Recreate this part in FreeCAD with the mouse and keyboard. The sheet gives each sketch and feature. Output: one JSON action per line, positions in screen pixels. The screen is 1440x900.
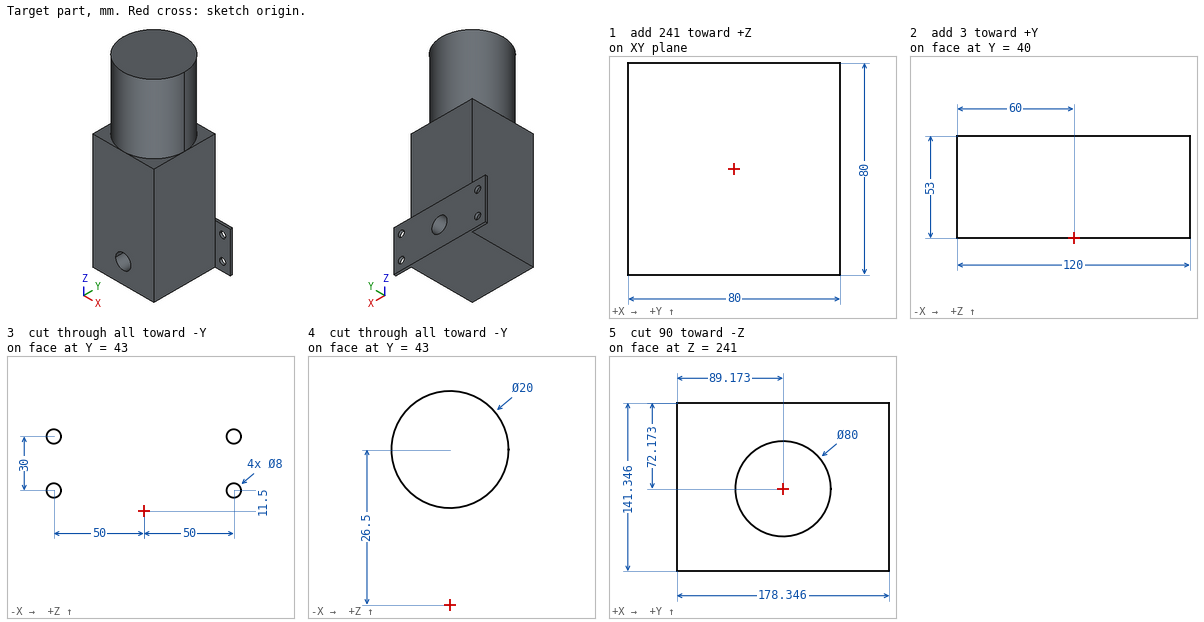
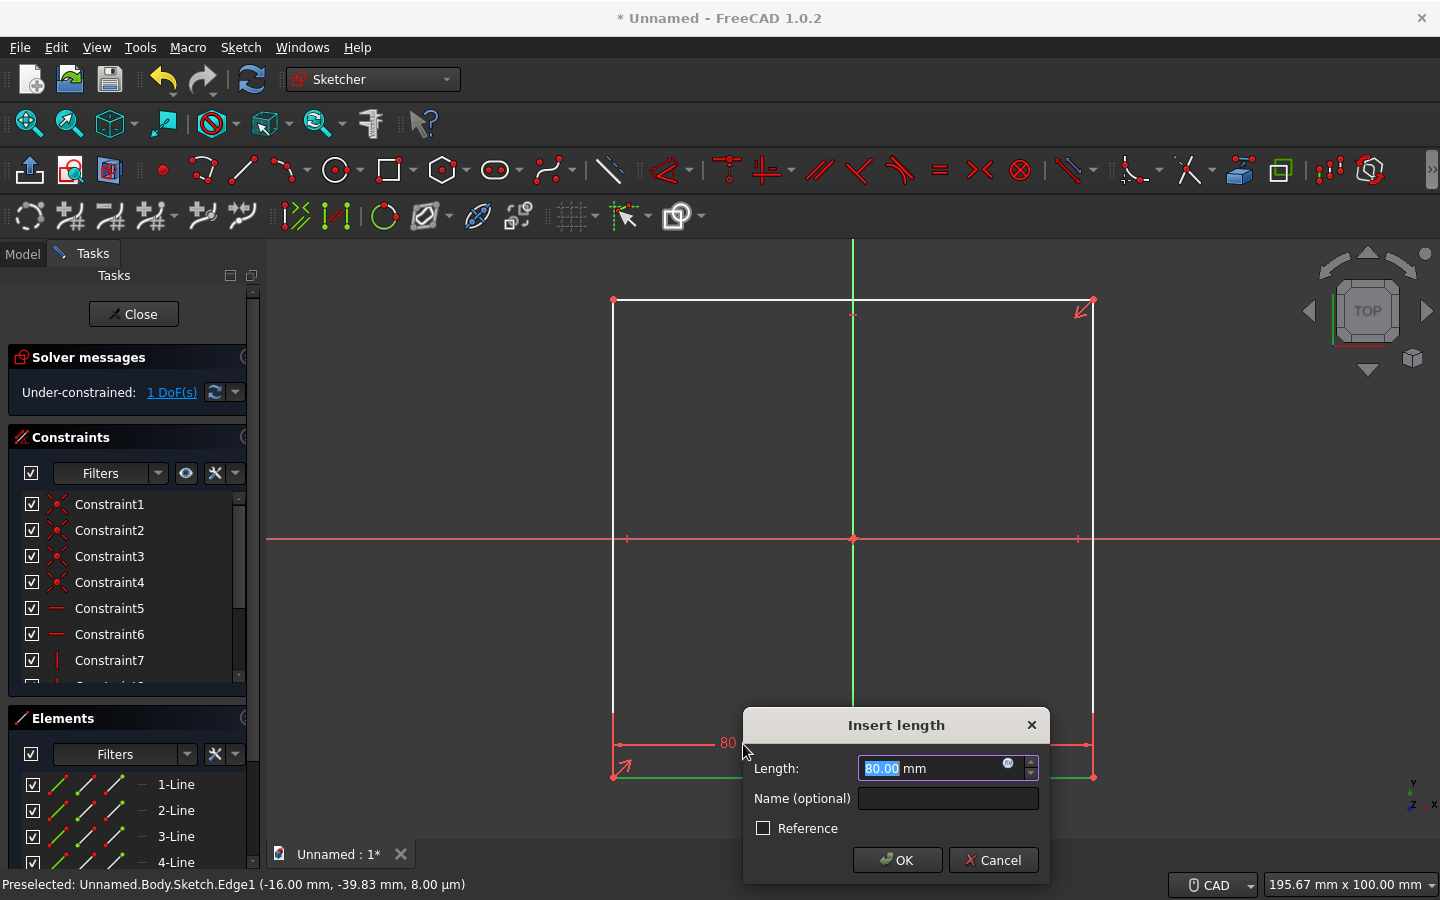
{"action": "type", "text": "80"}
{"action": "key", "text": "Return"}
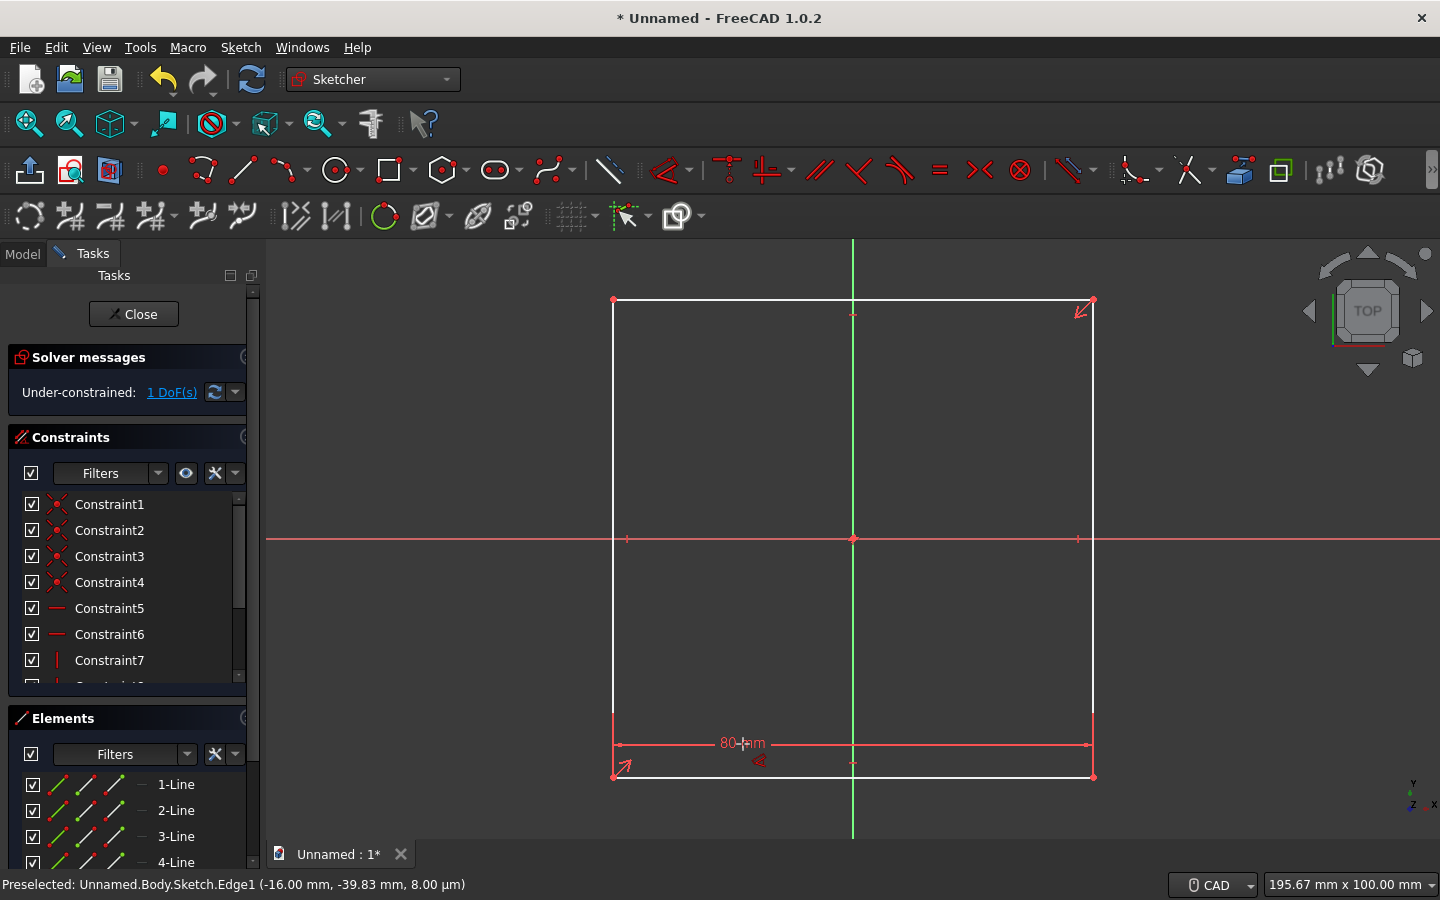
{"action": "left_click", "coordinate": [1093, 635]}
{"action": "left_click", "coordinate": [1127, 429]}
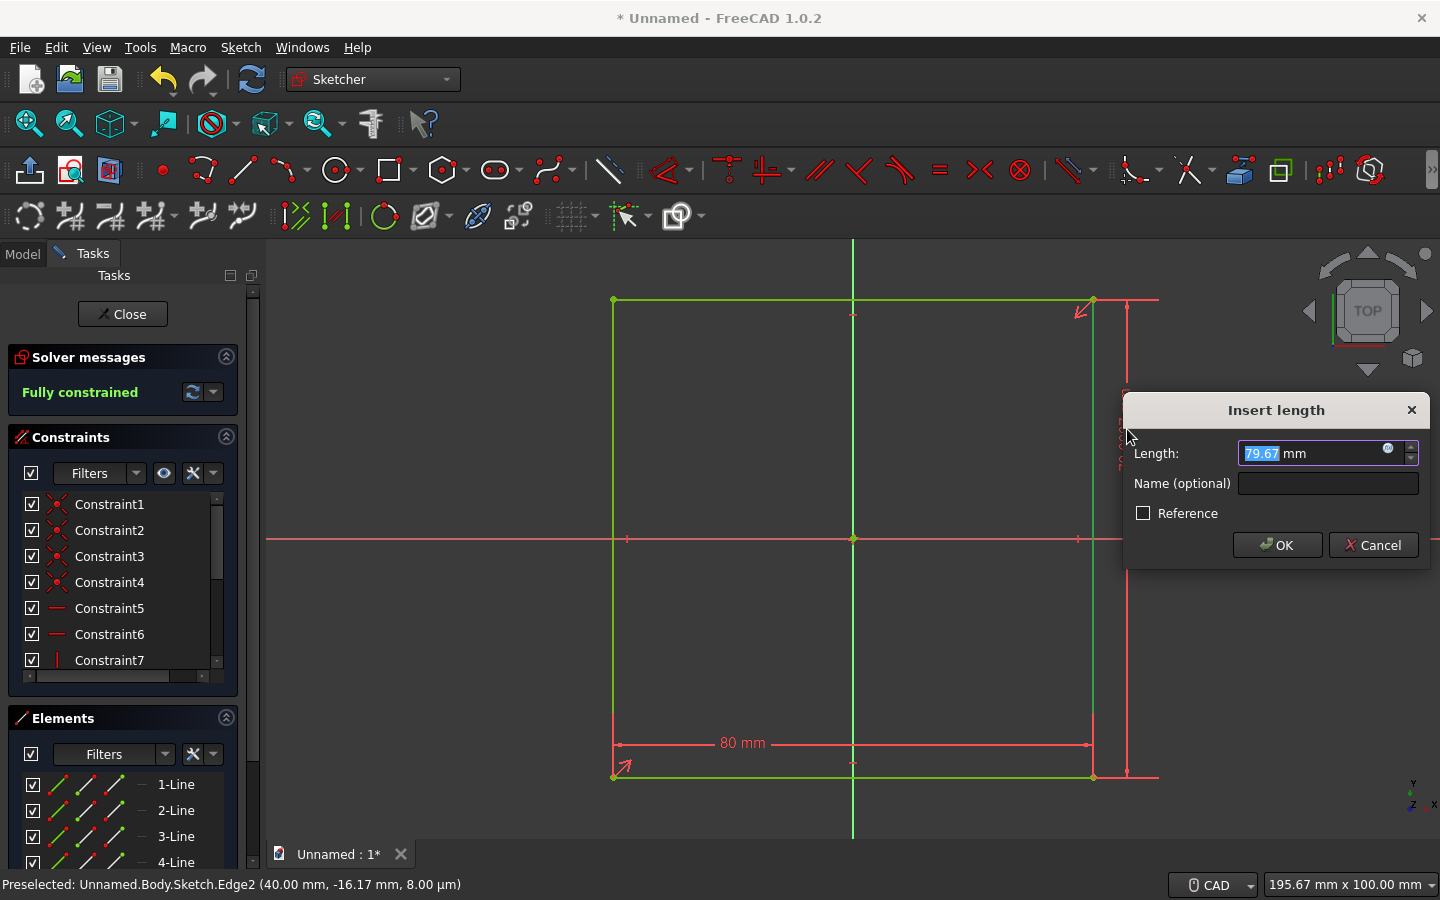
{"action": "type", "text": "80"}
{"action": "key", "text": "Return"}
{"action": "key", "text": "Escape"}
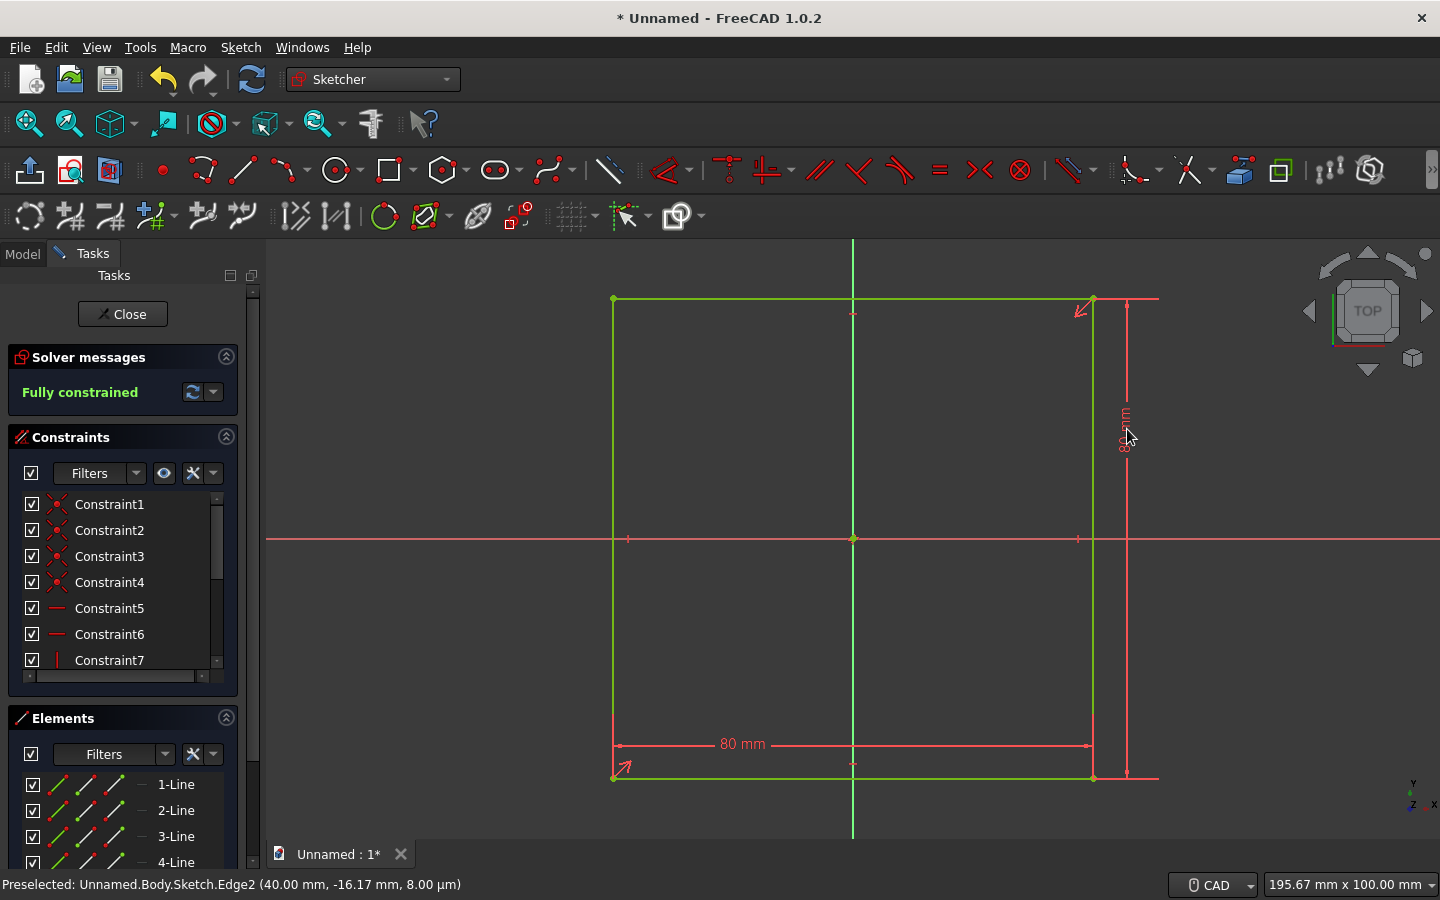
{"action": "left_click", "coordinate": [123, 314]}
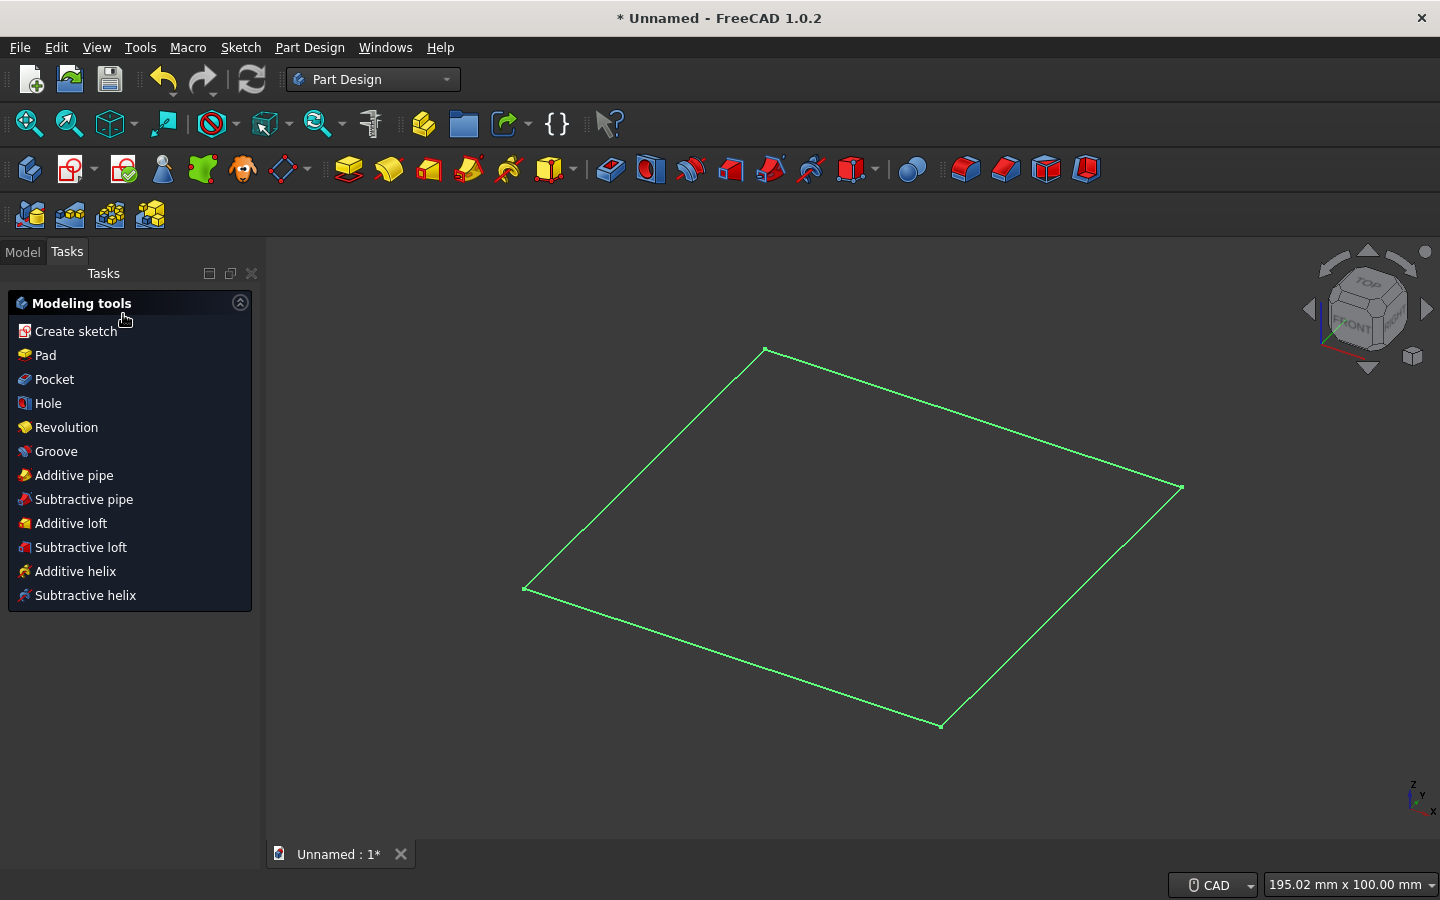
{"action": "left_click", "coordinate": [350, 170]}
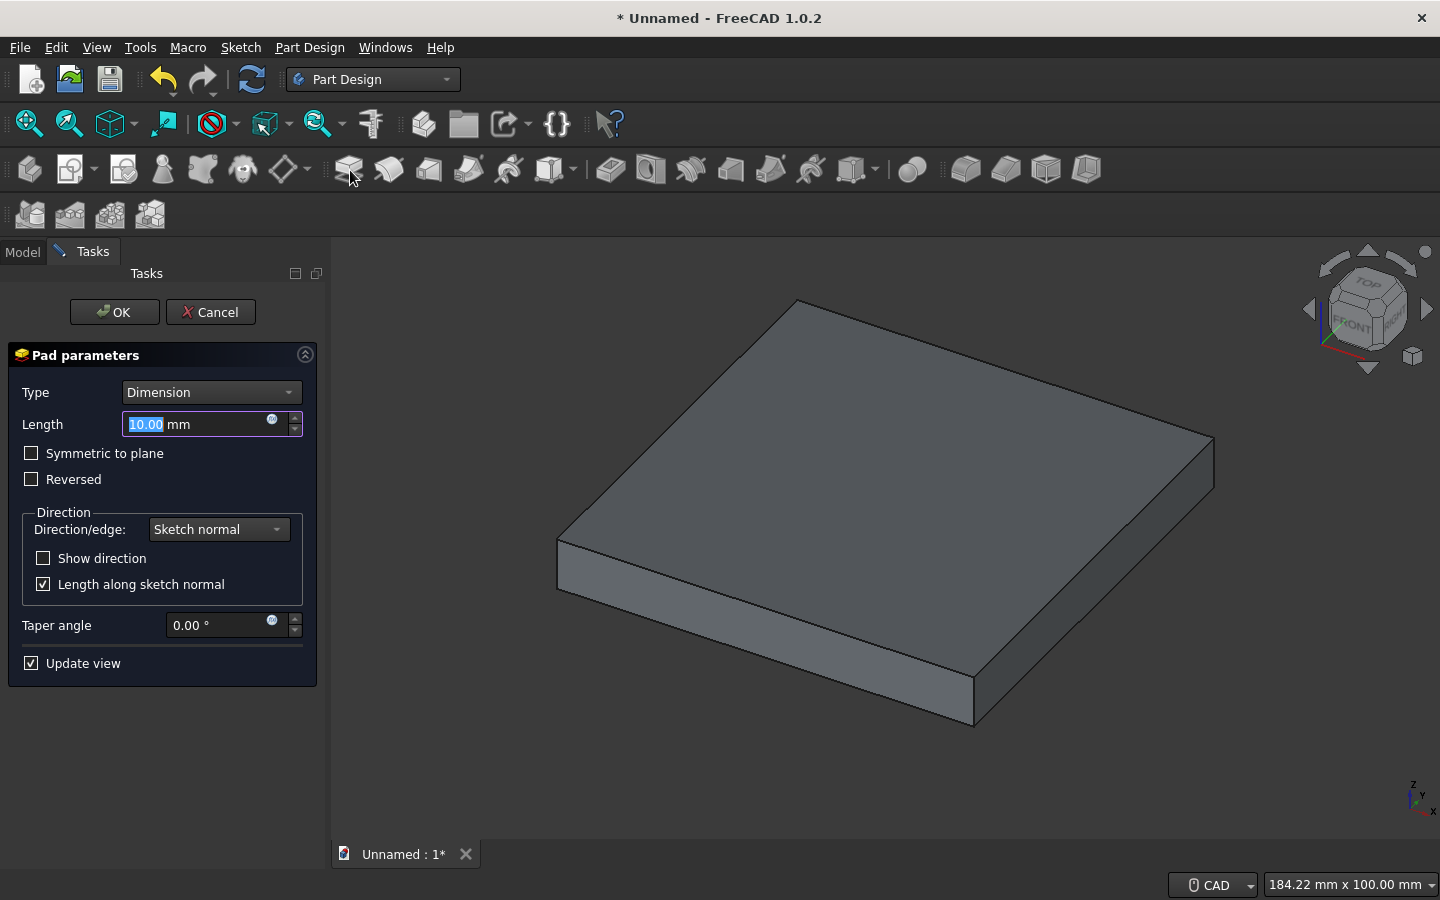
{"action": "type", "text": "241"}
{"action": "key", "text": "Tab"}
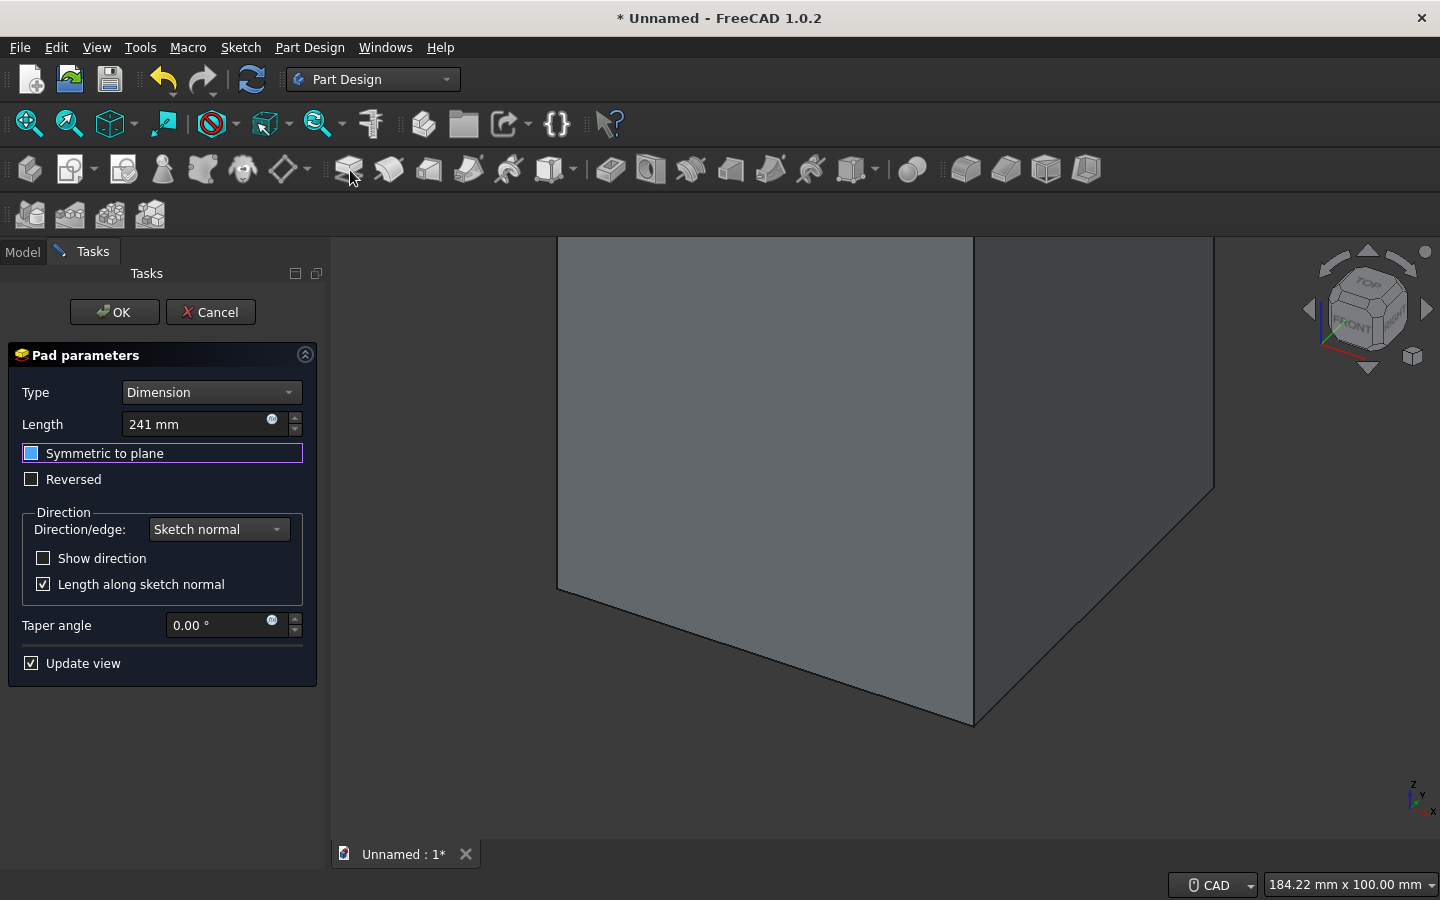
{"action": "left_click", "coordinate": [115, 312]}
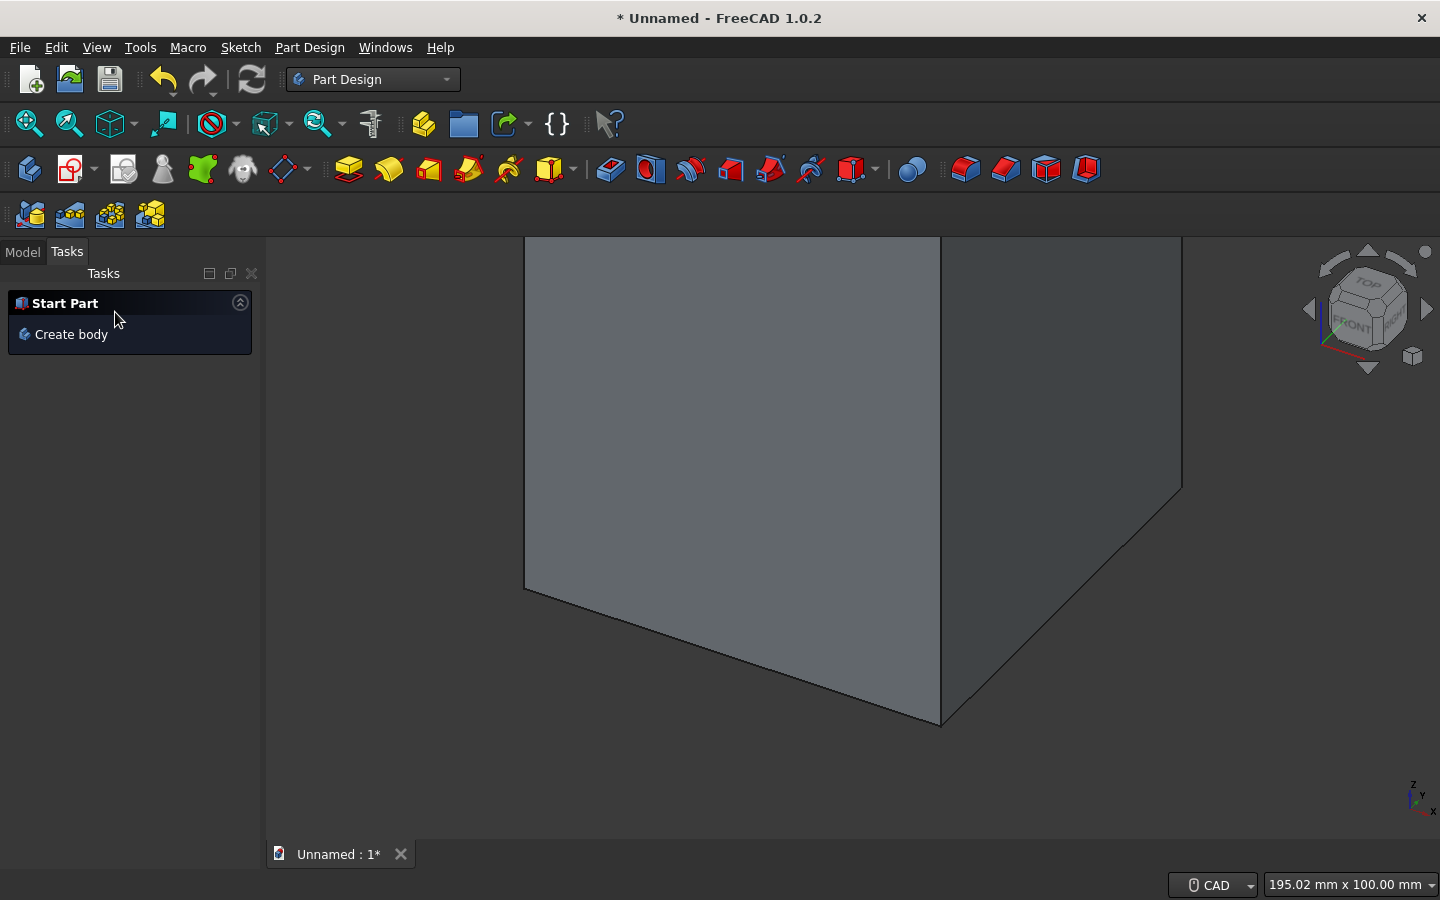
{"action": "left_click", "coordinate": [30, 124]}